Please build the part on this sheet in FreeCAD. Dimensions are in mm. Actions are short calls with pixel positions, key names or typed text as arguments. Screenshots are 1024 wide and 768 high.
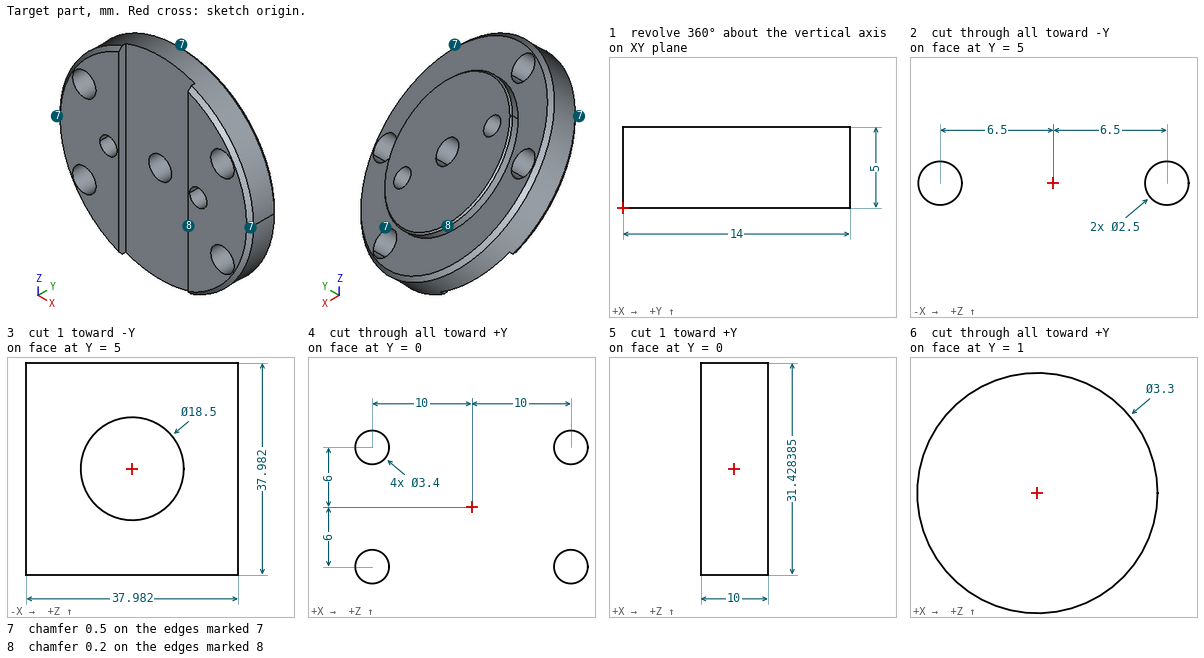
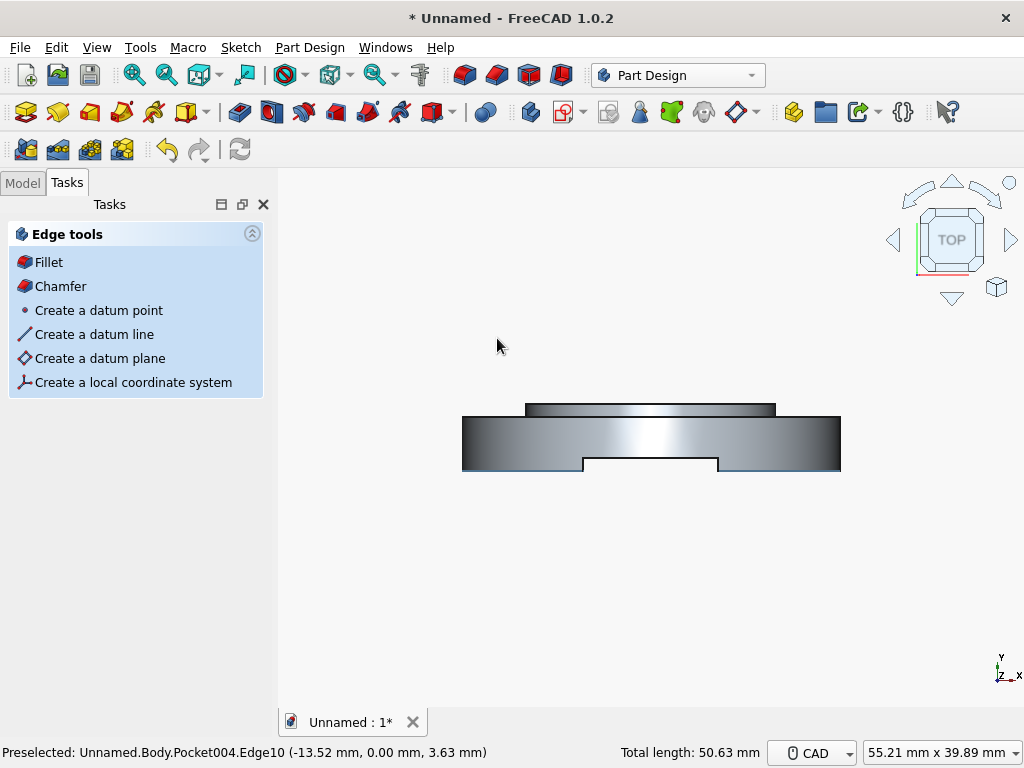
click(709, 416, ctrl)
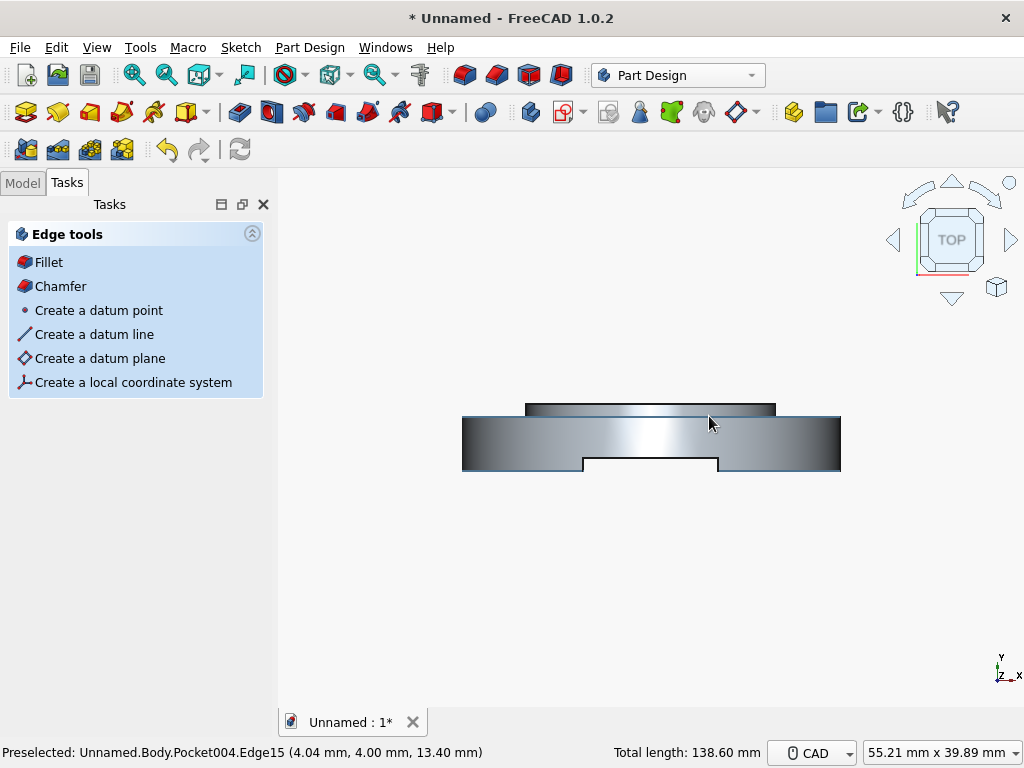
click(498, 76)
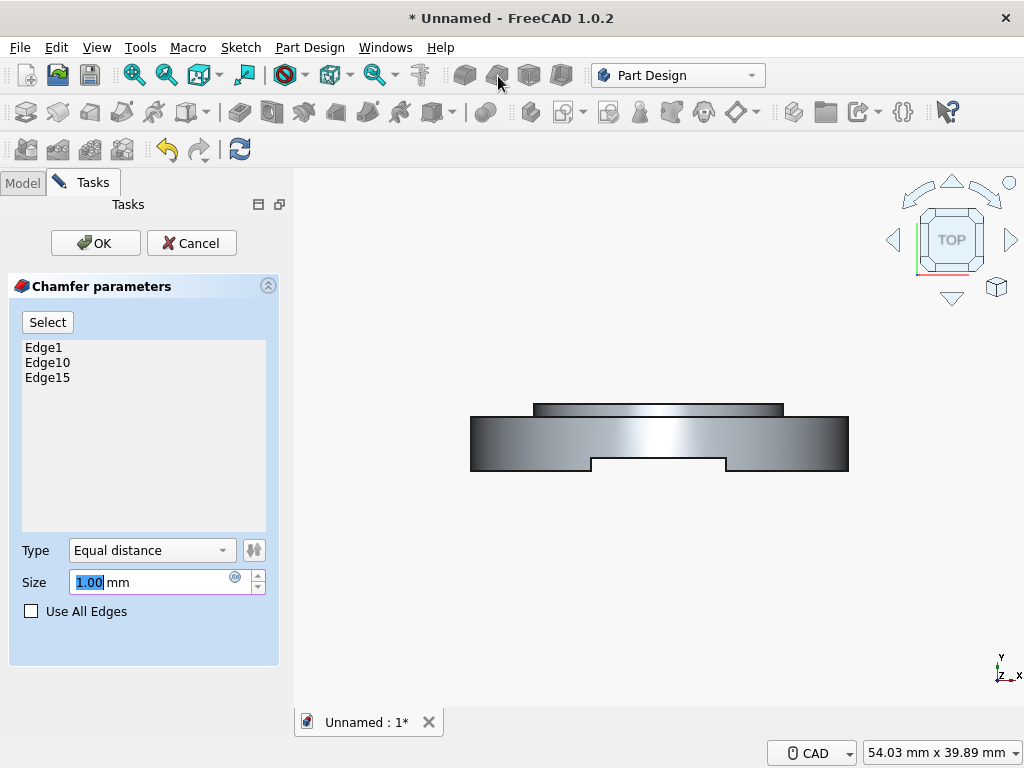
text(0.5)
key(Tab)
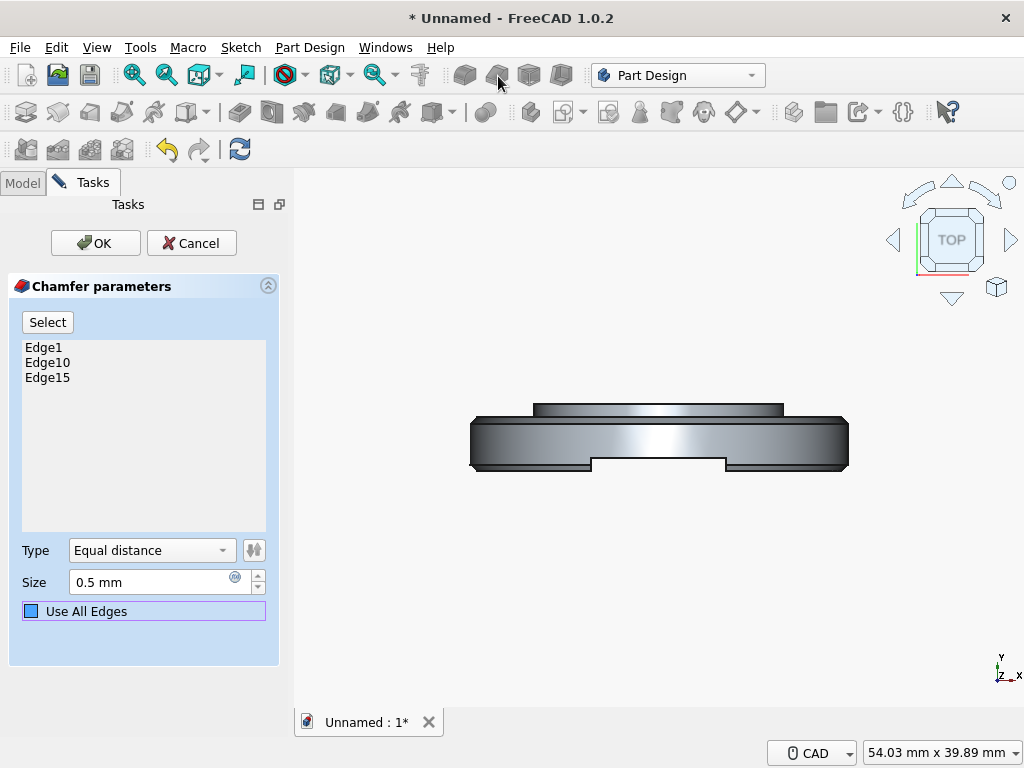
click(96, 243)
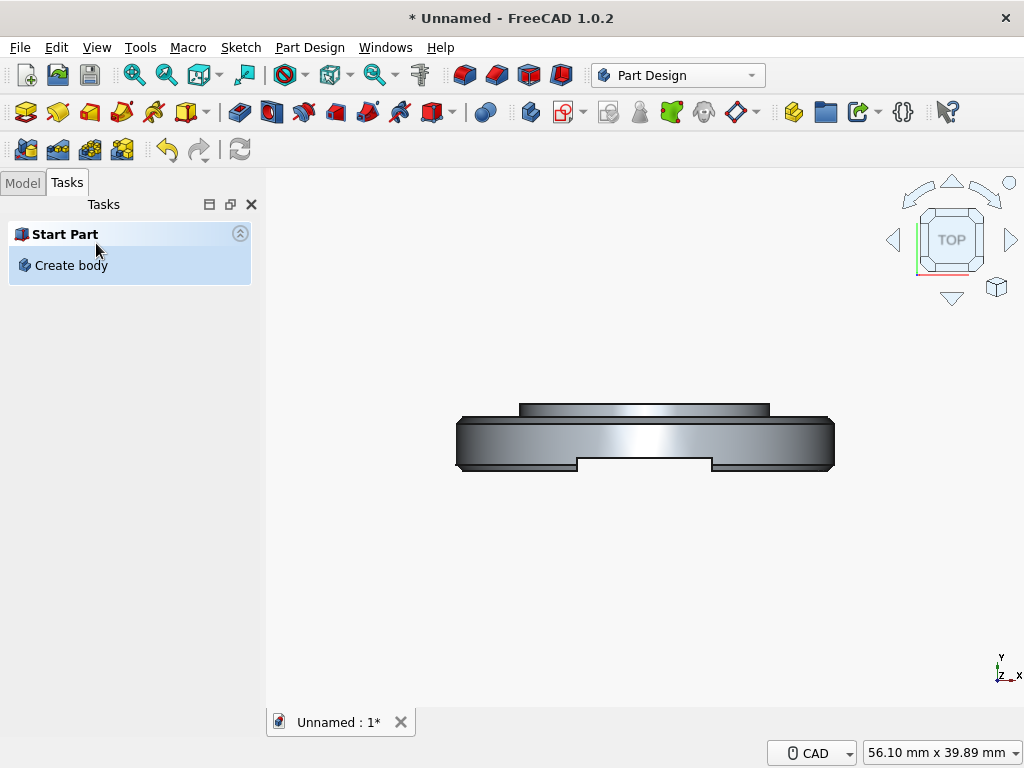
click(746, 403)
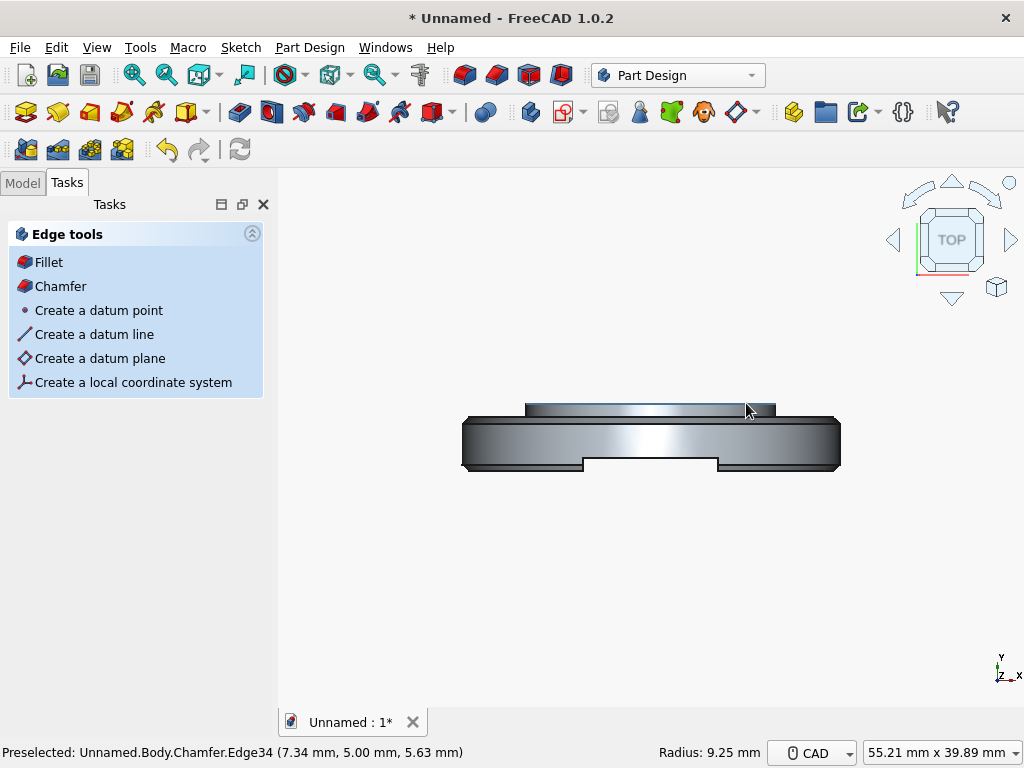
click(498, 76)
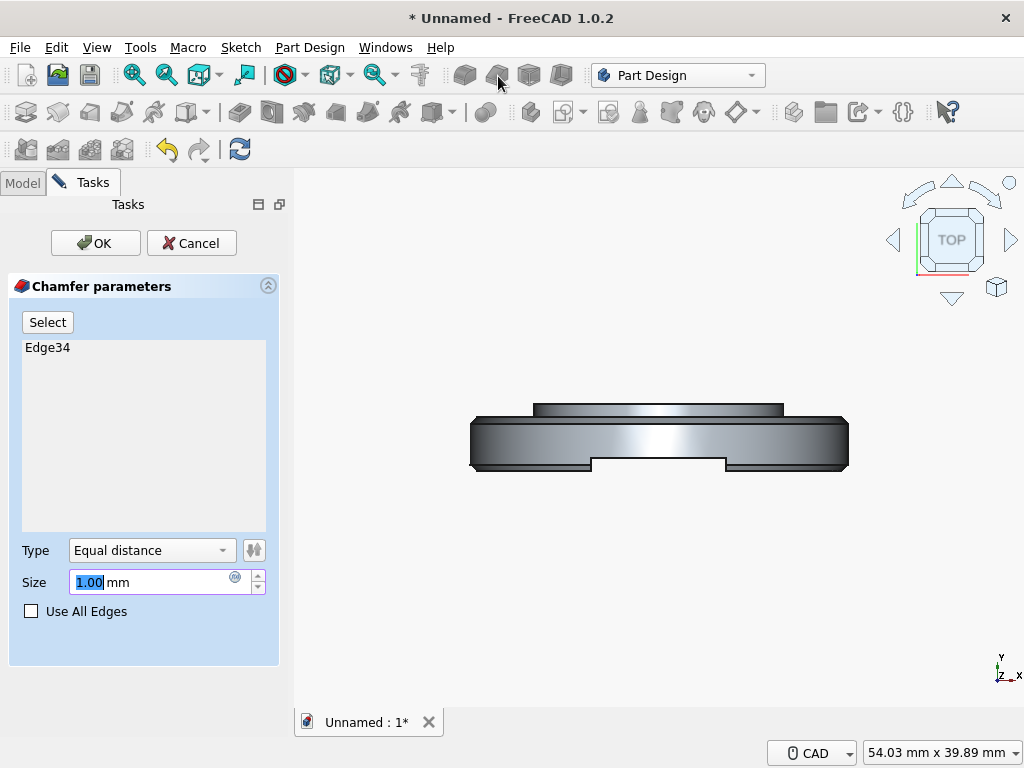
text(0.2)
key(Tab)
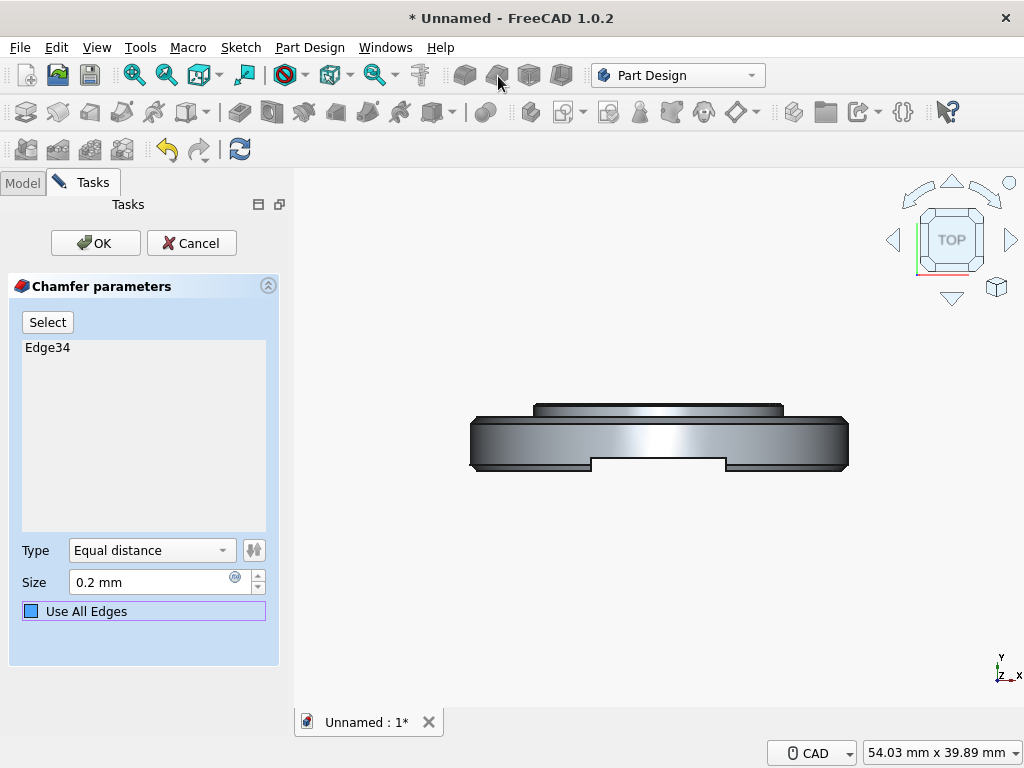
click(96, 243)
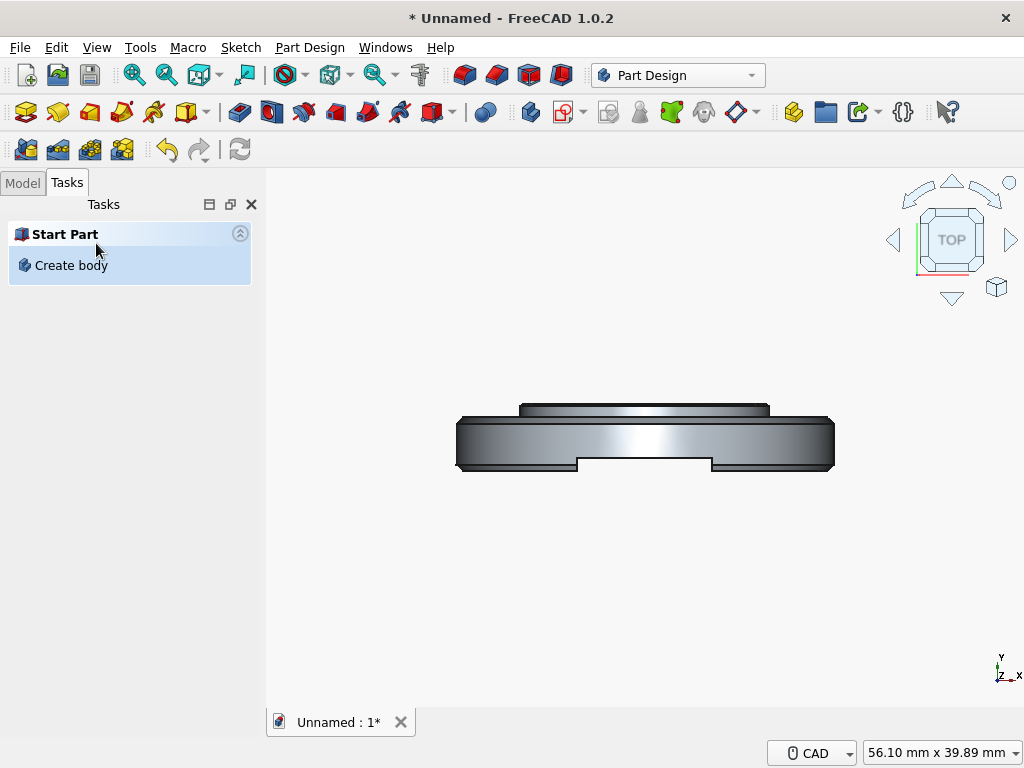
key(0)